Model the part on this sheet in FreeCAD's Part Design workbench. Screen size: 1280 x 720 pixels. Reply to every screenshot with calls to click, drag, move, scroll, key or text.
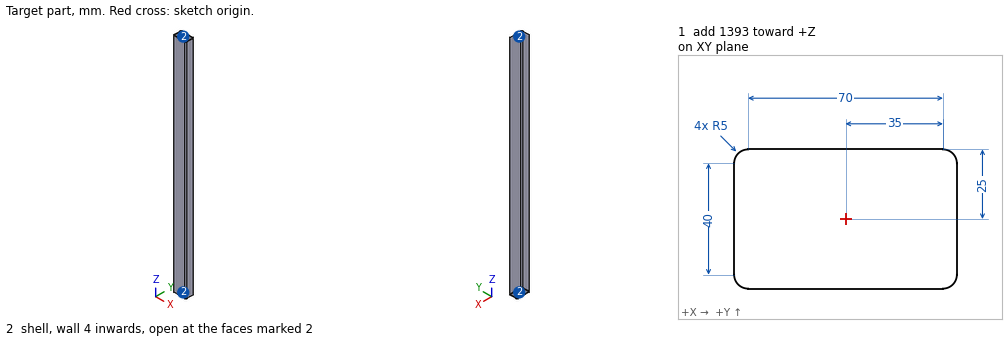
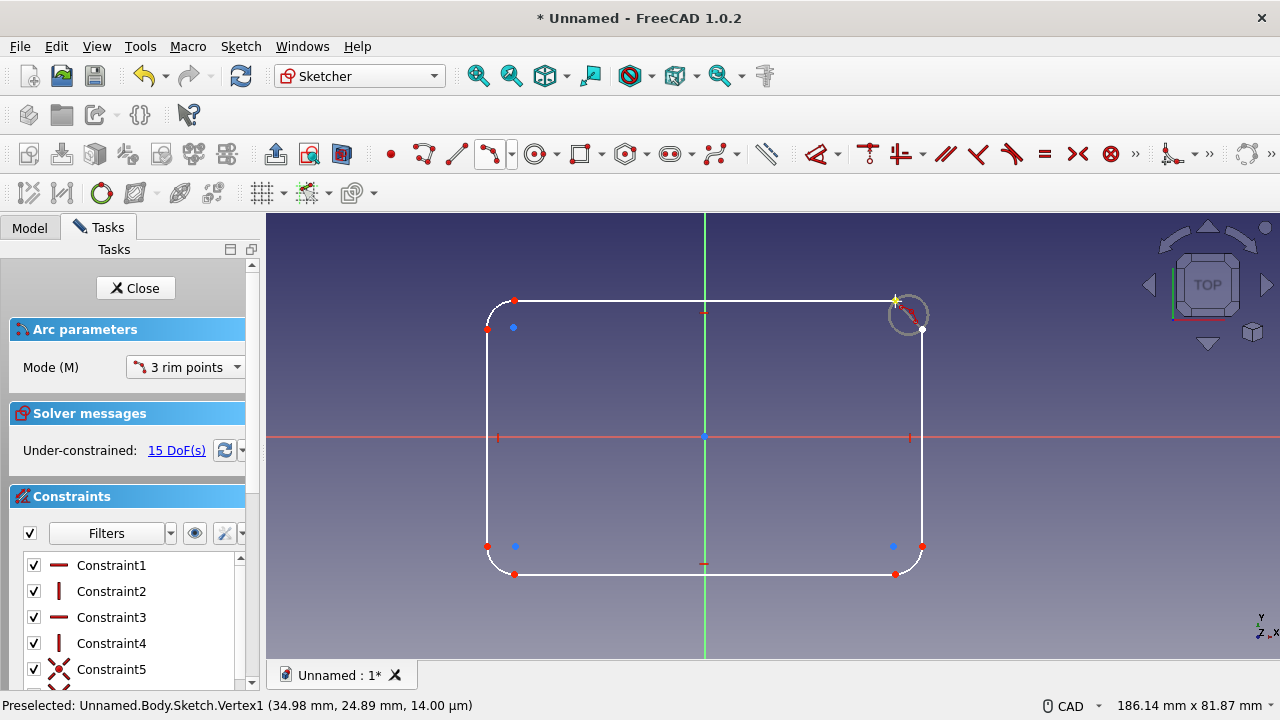
scroll(915, 308, up, 4)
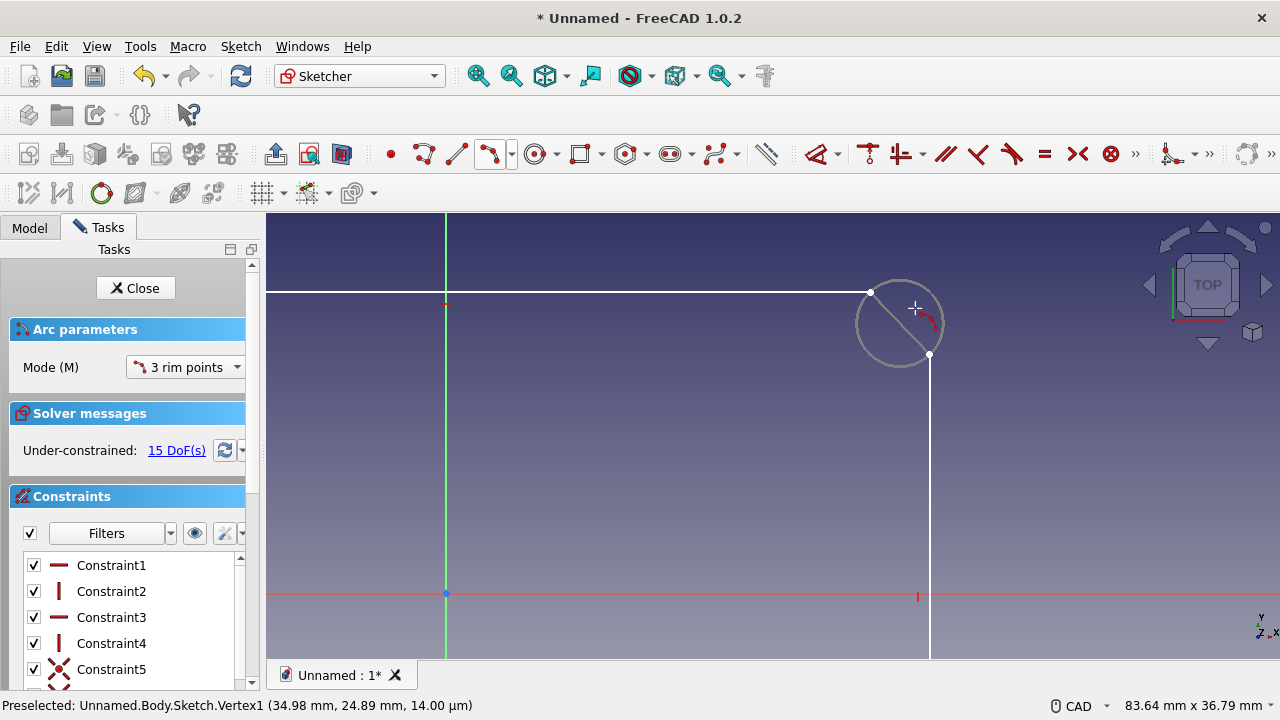
click(913, 309)
key(Escape)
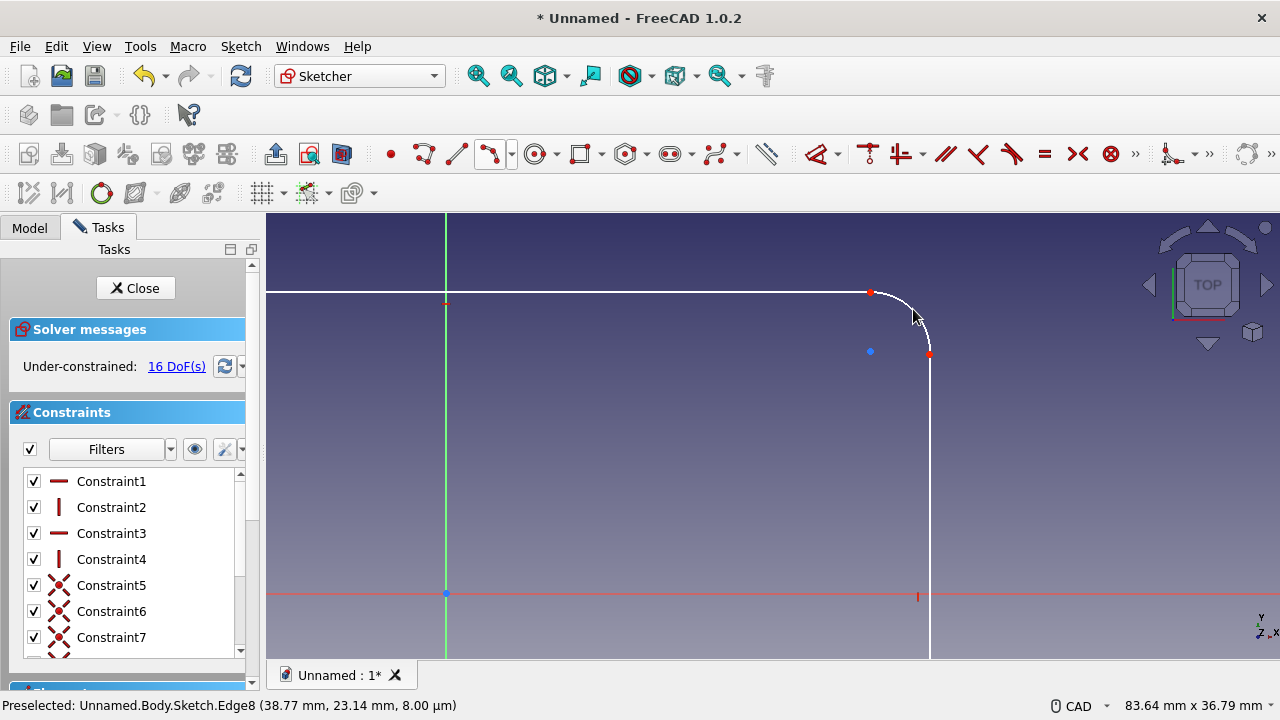
click(616, 292)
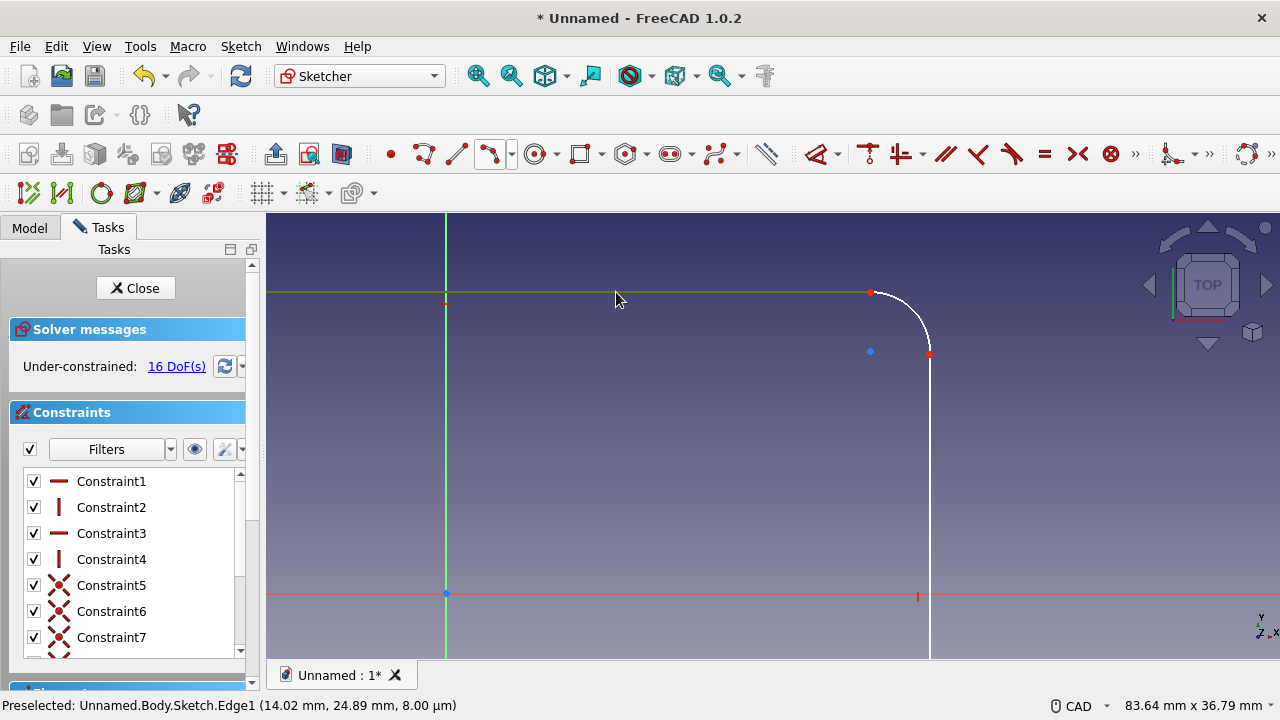
scroll(915, 307, down, 4)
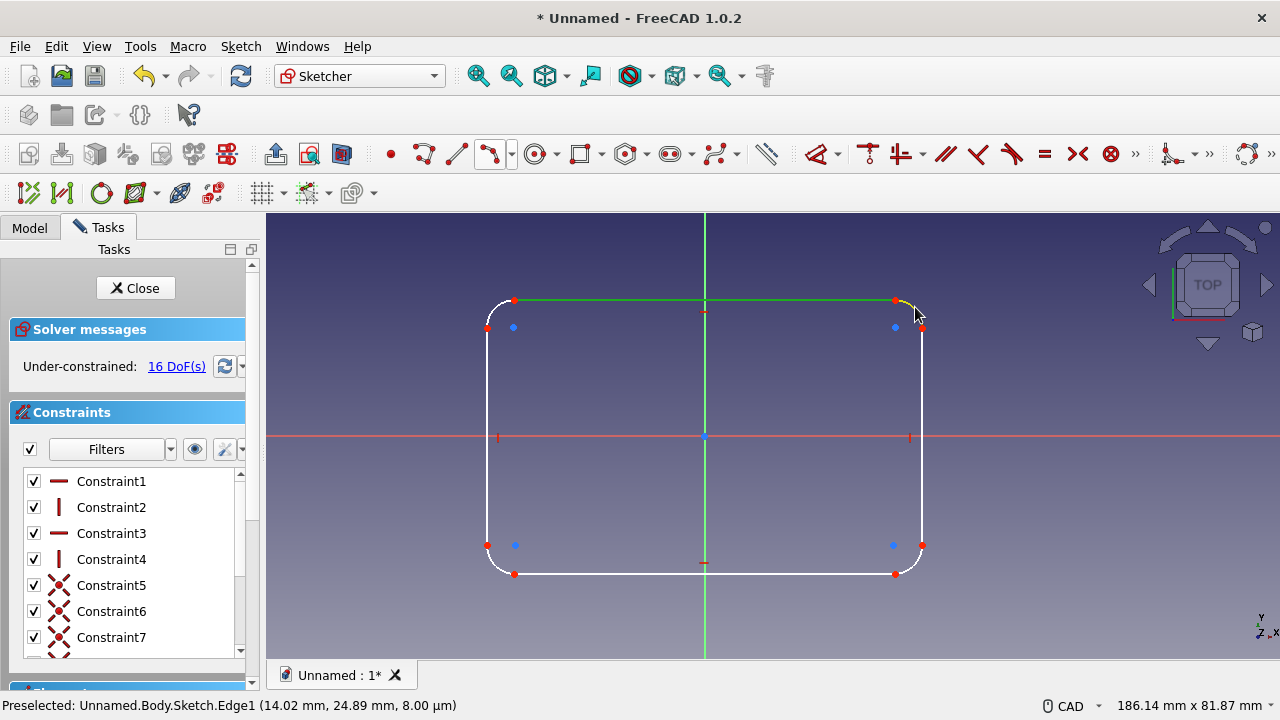
click(502, 303)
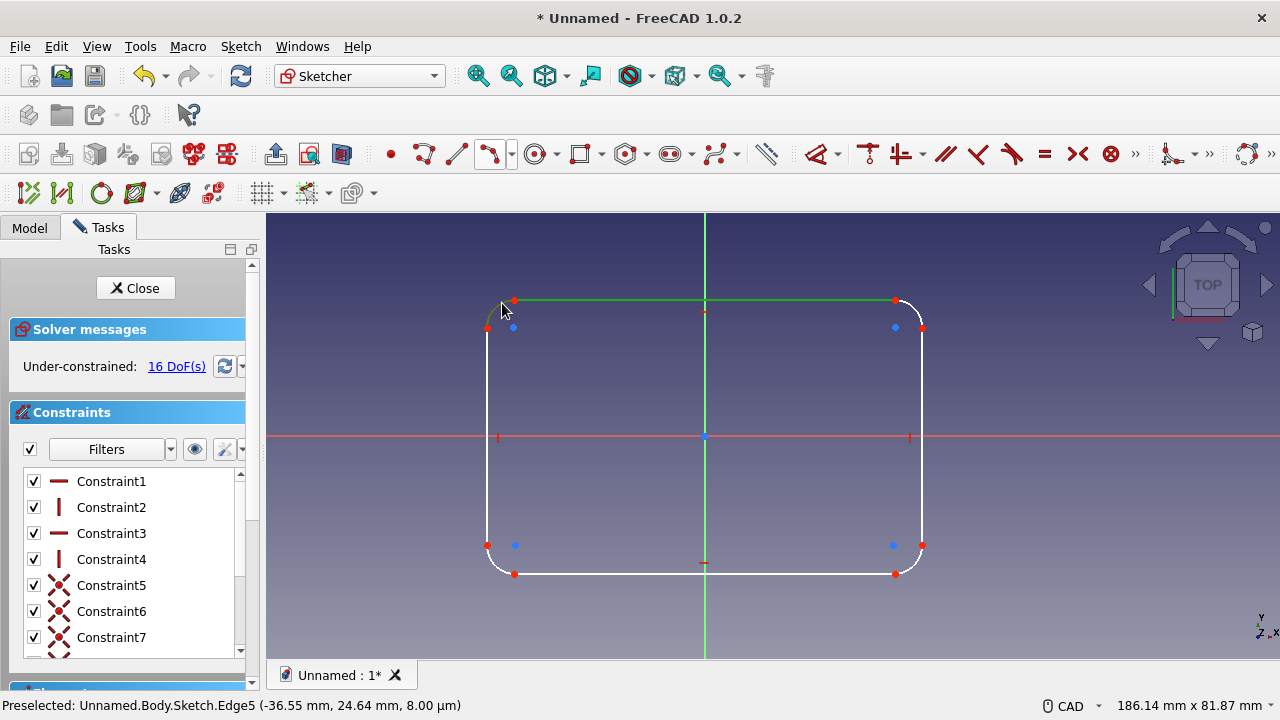
click(1012, 154)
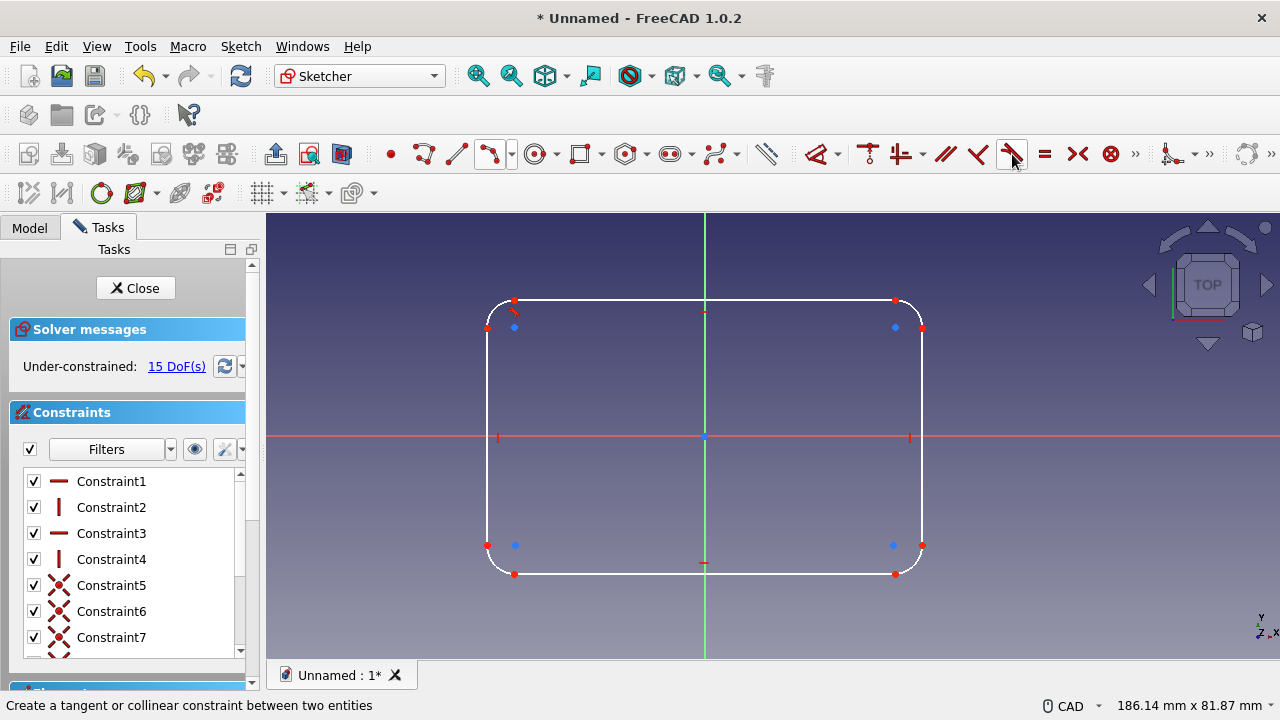
click(781, 300)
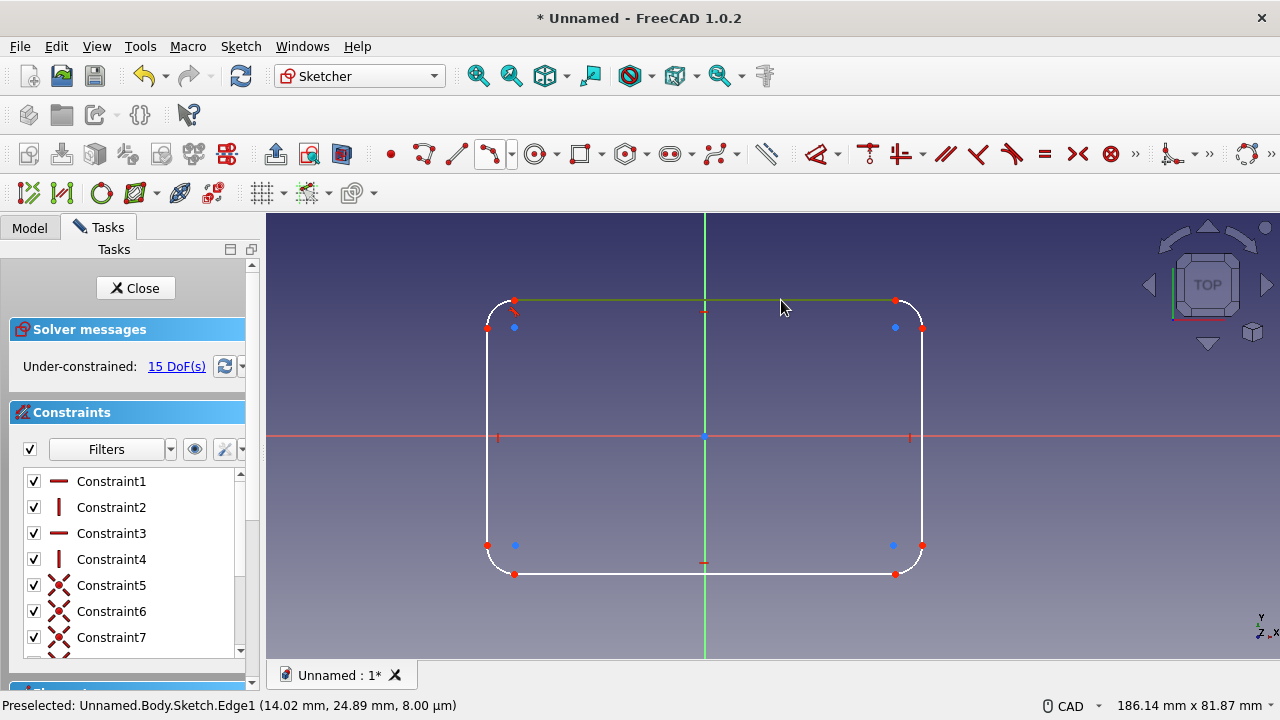
click(920, 316)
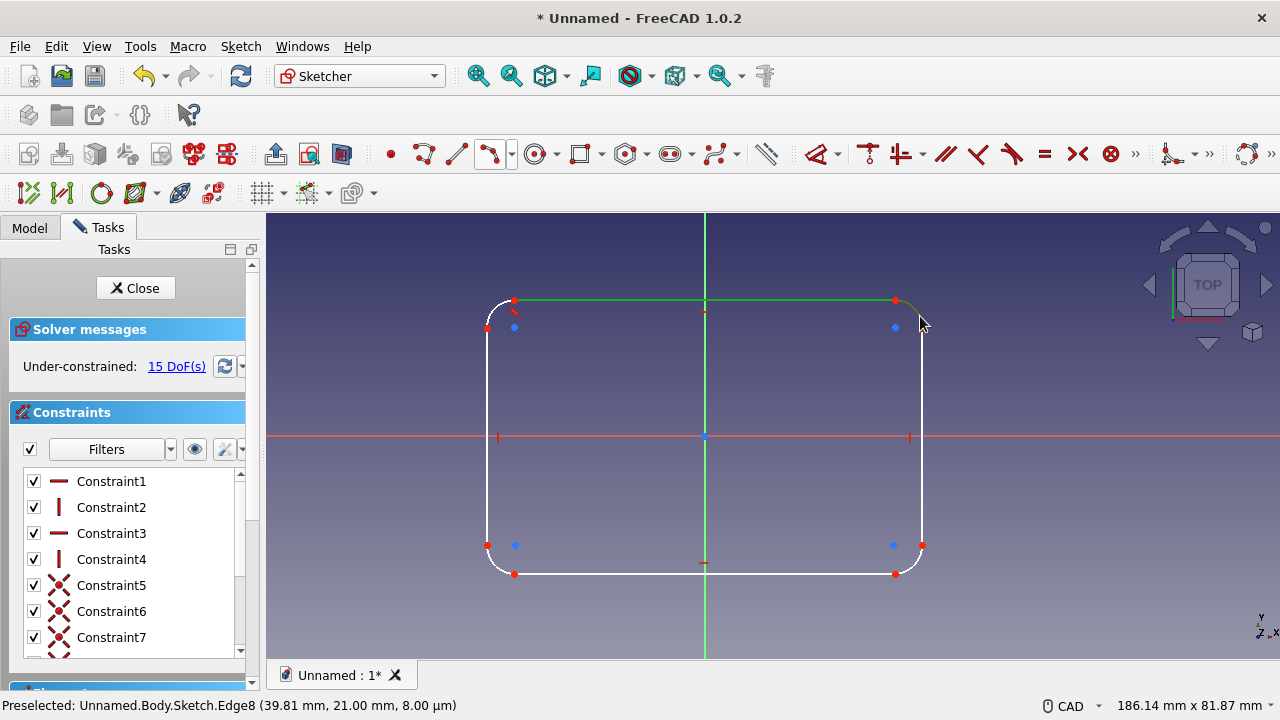
click(1012, 154)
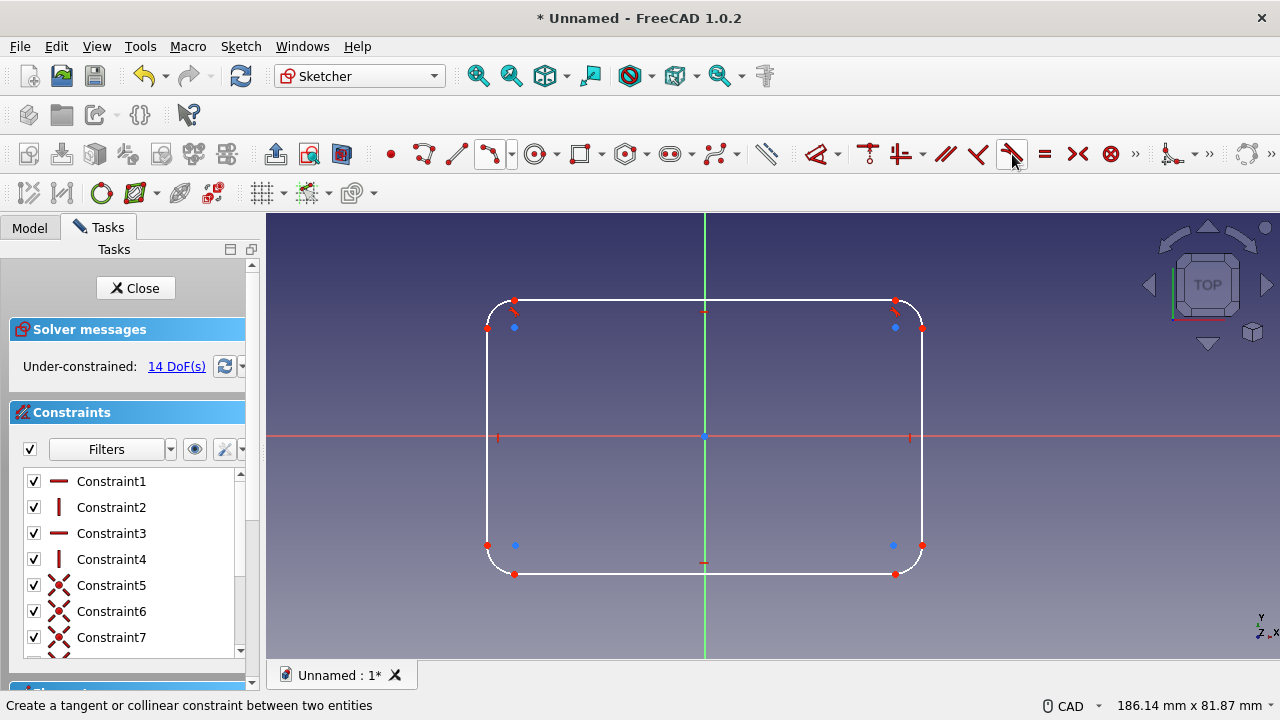
click(487, 394)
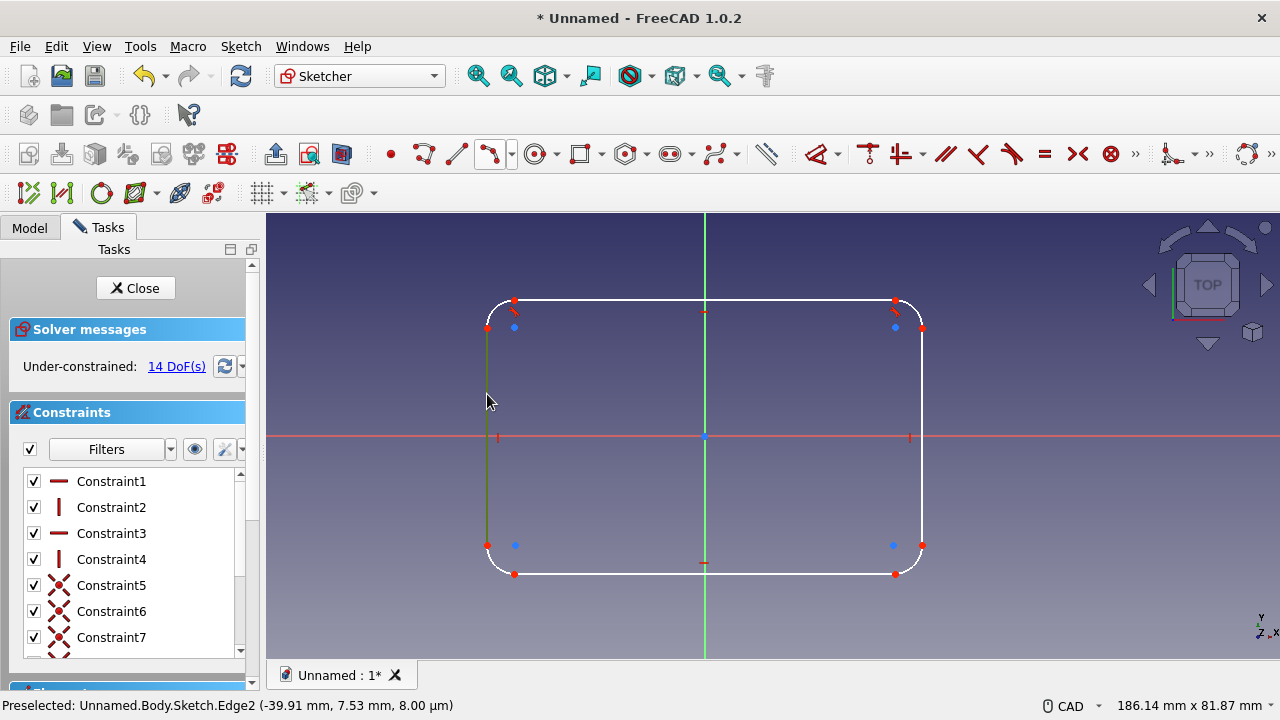
click(502, 304)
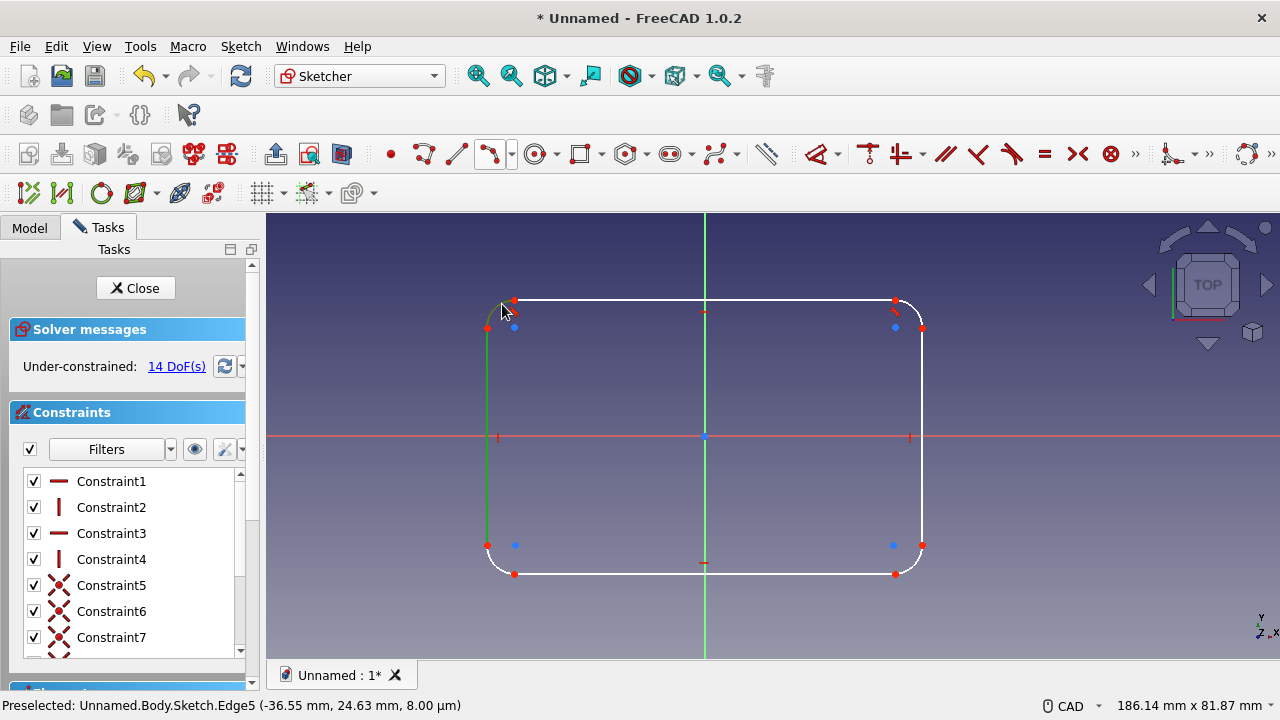
click(1012, 154)